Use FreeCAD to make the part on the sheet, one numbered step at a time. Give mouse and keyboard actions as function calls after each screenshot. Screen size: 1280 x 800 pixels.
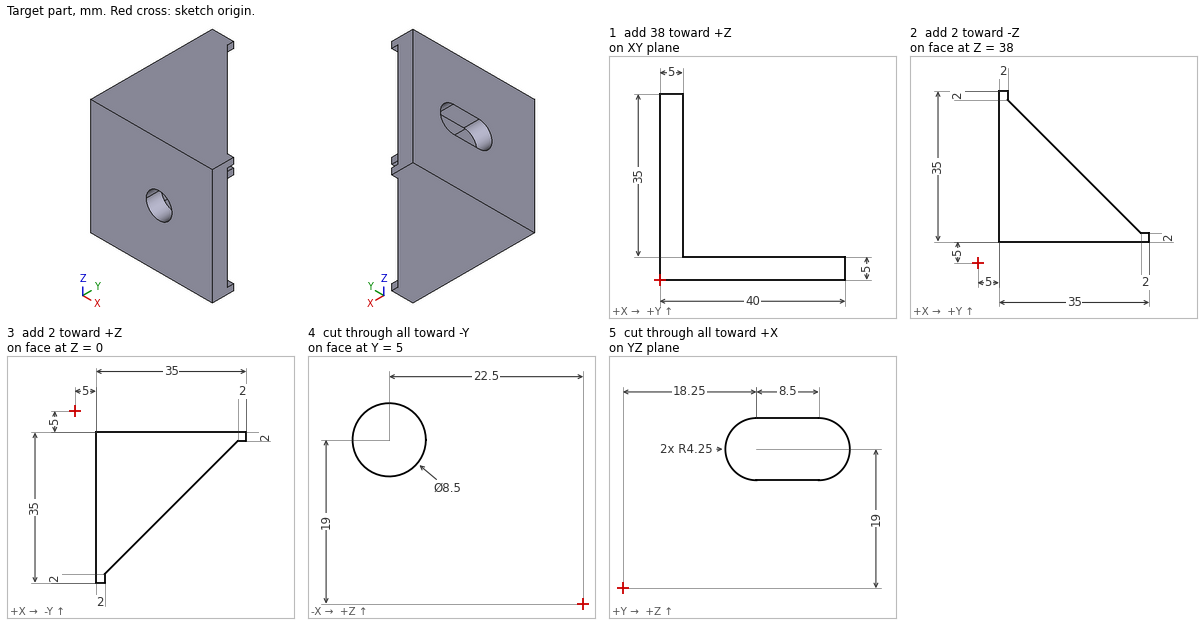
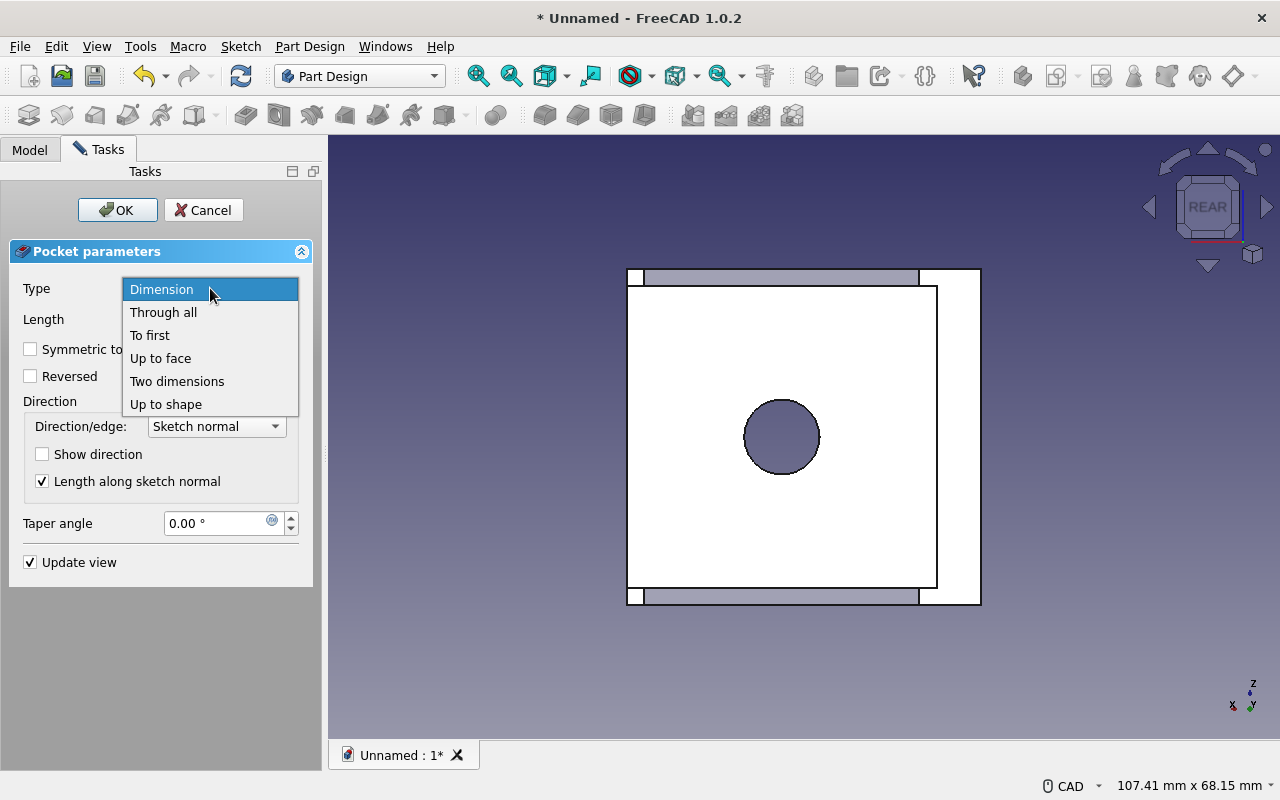
click(208, 312)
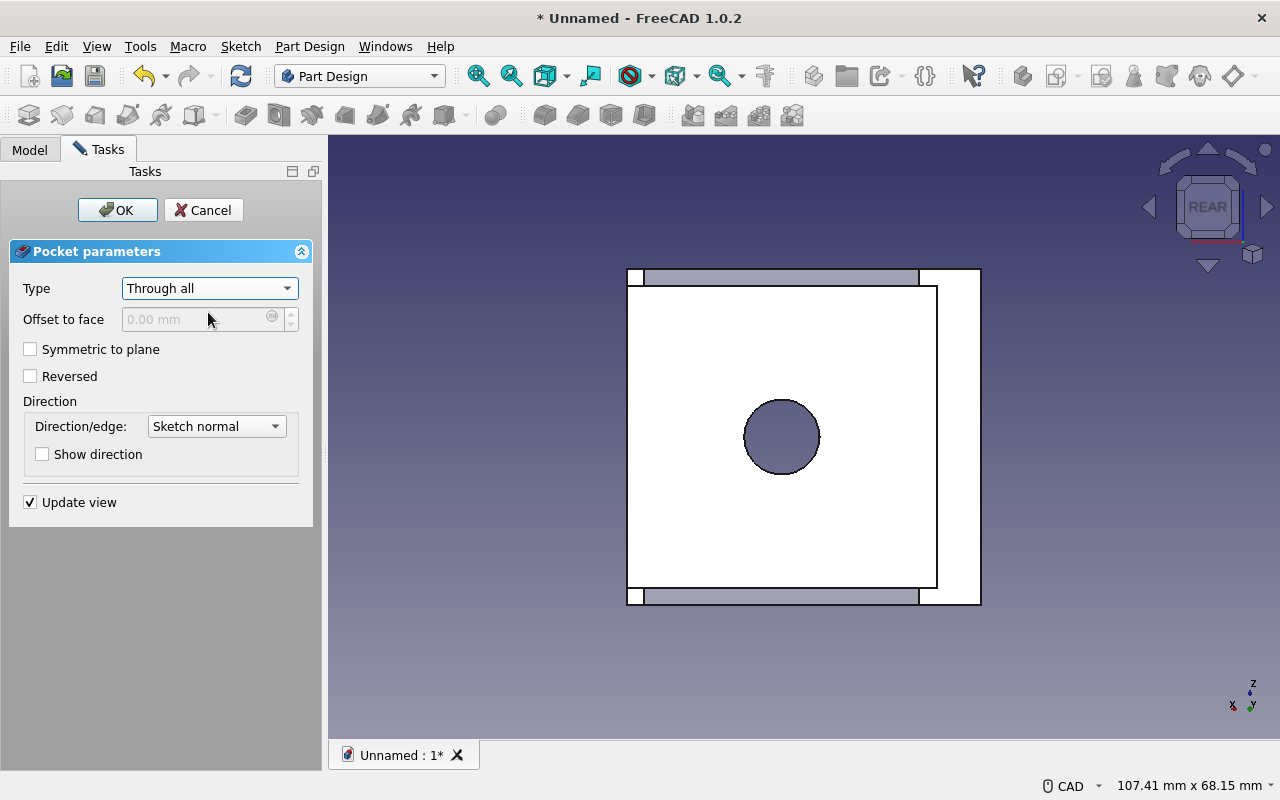
click(31, 376)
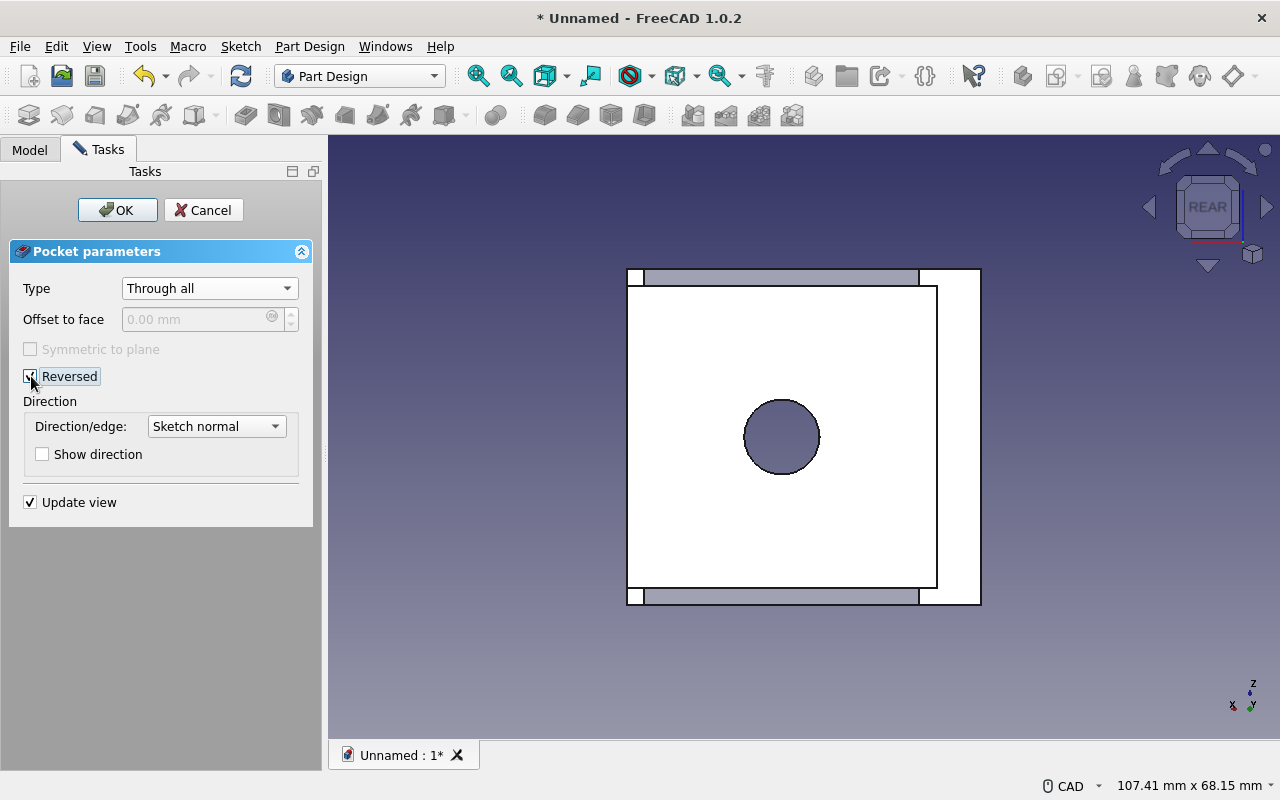
click(118, 210)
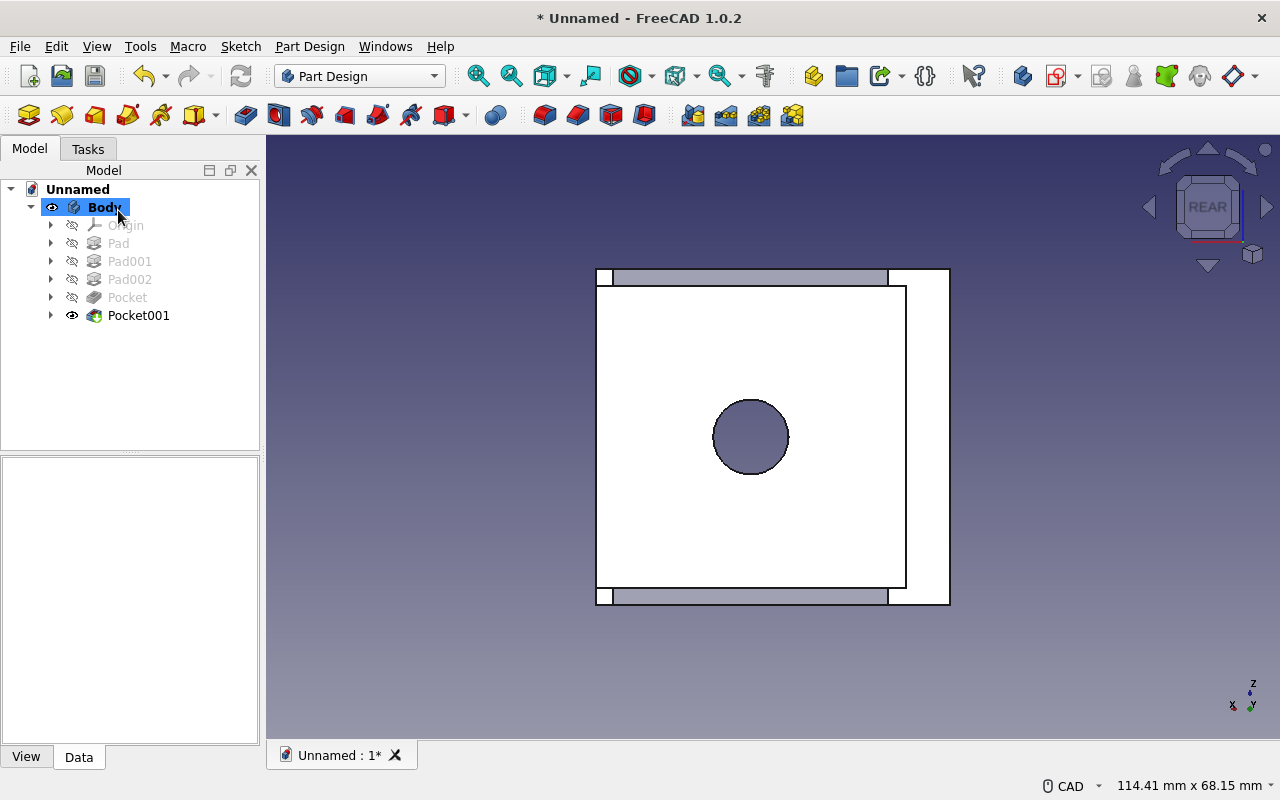
key(0)